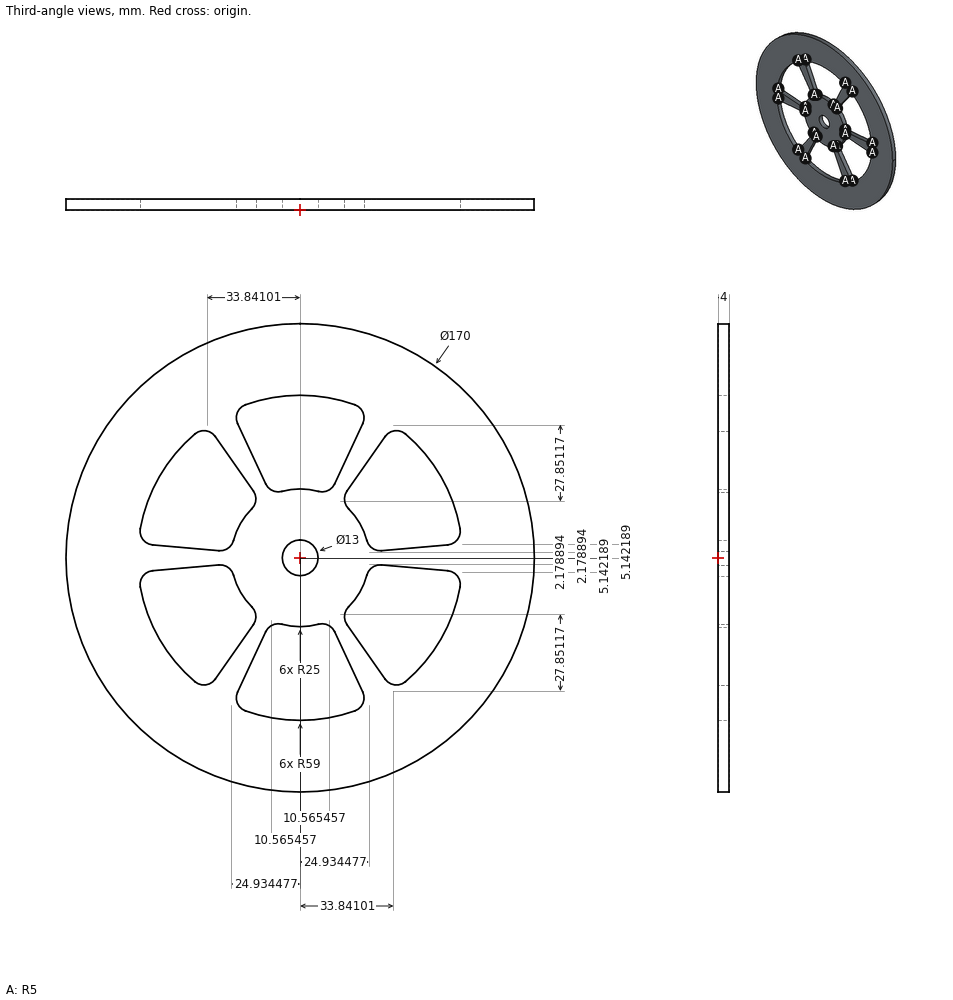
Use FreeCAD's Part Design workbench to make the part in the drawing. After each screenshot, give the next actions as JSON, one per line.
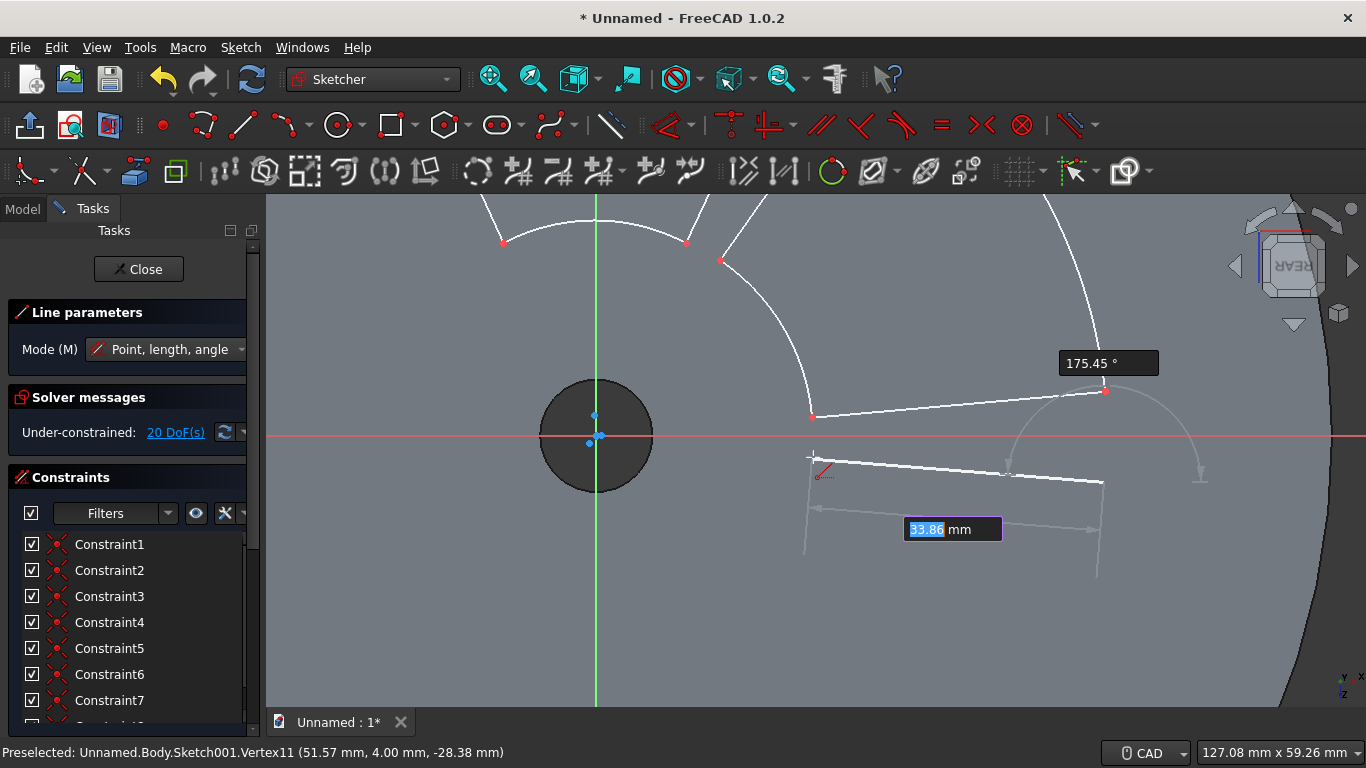
{"action": "left_click", "coordinate": [812, 455]}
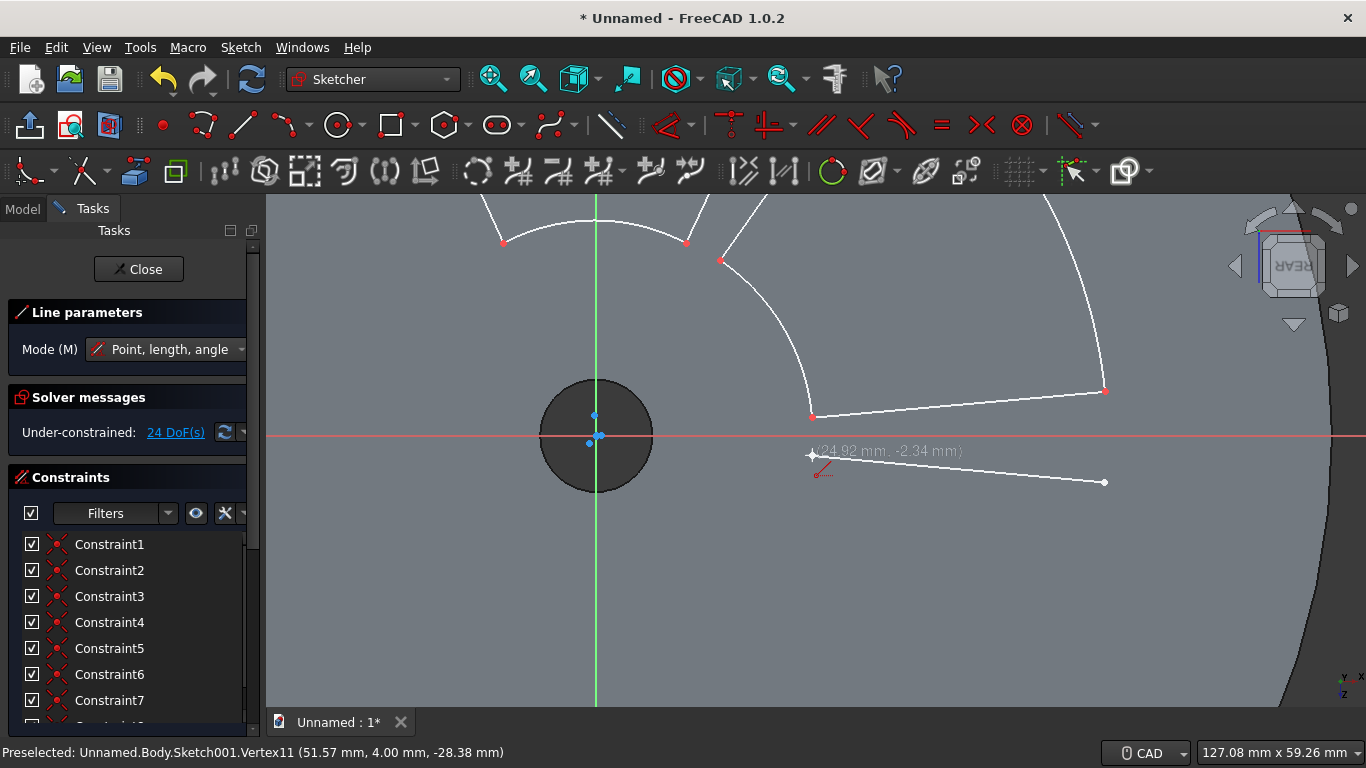
{"action": "scroll", "coordinate": [813, 457], "scroll_direction": "down", "scroll_amount": 6}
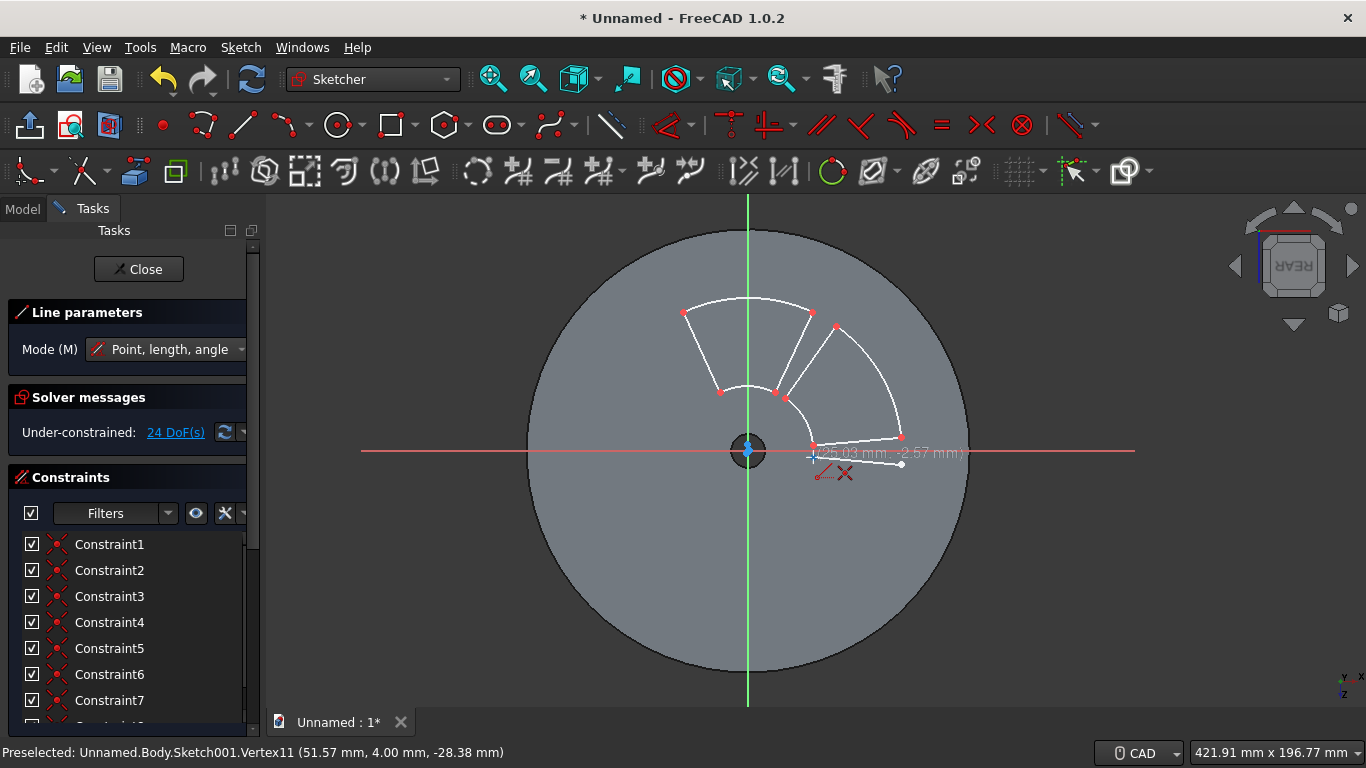
{"action": "left_click", "coordinate": [785, 504]}
{"action": "left_click", "coordinate": [836, 577]}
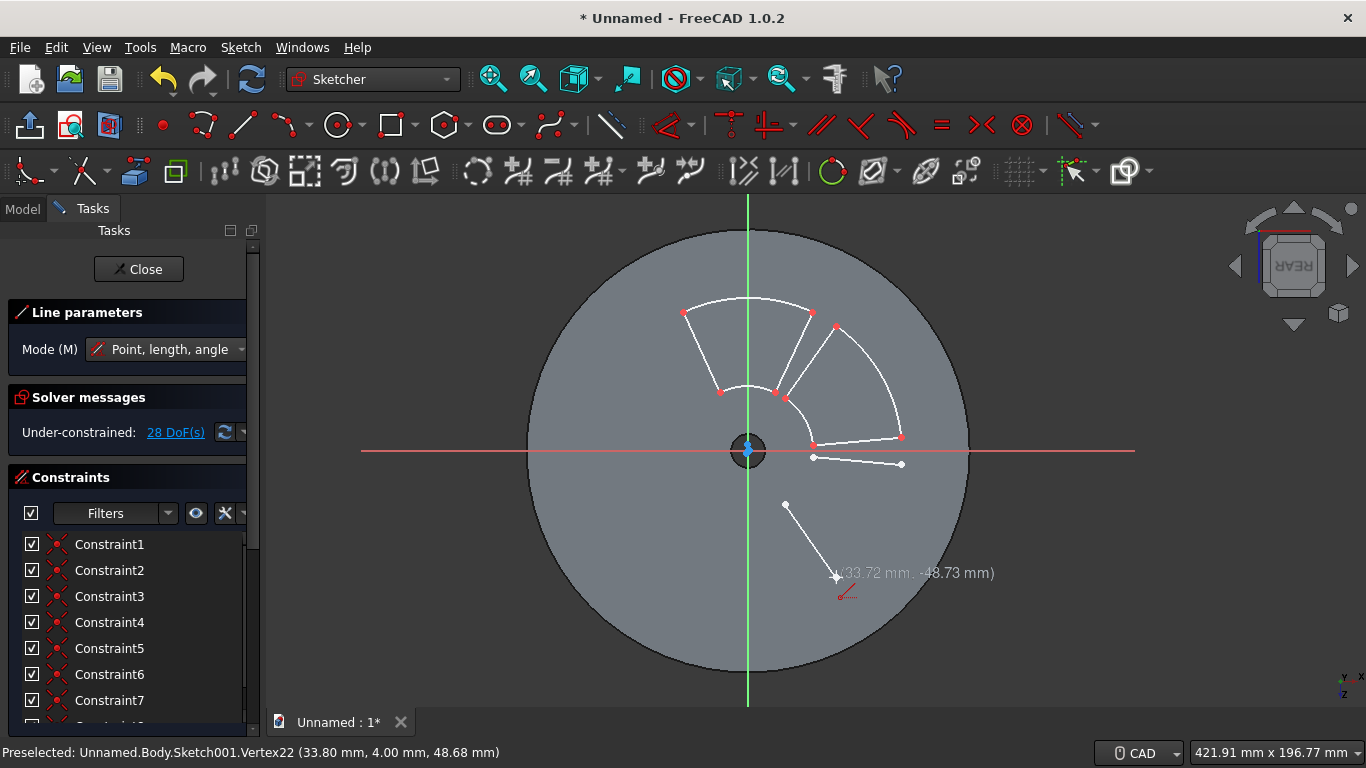
{"action": "left_click", "coordinate": [284, 126]}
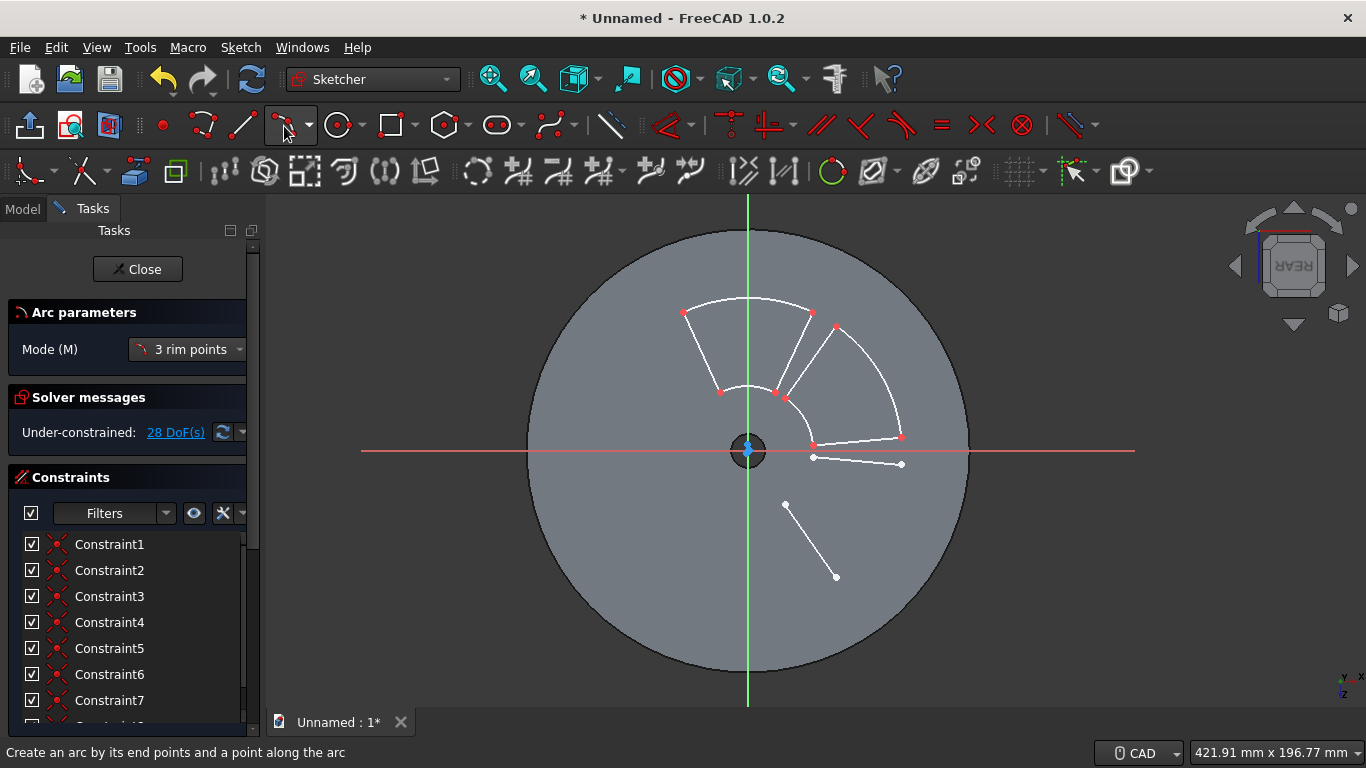
{"action": "scroll", "coordinate": [813, 457], "scroll_direction": "up", "scroll_amount": 6}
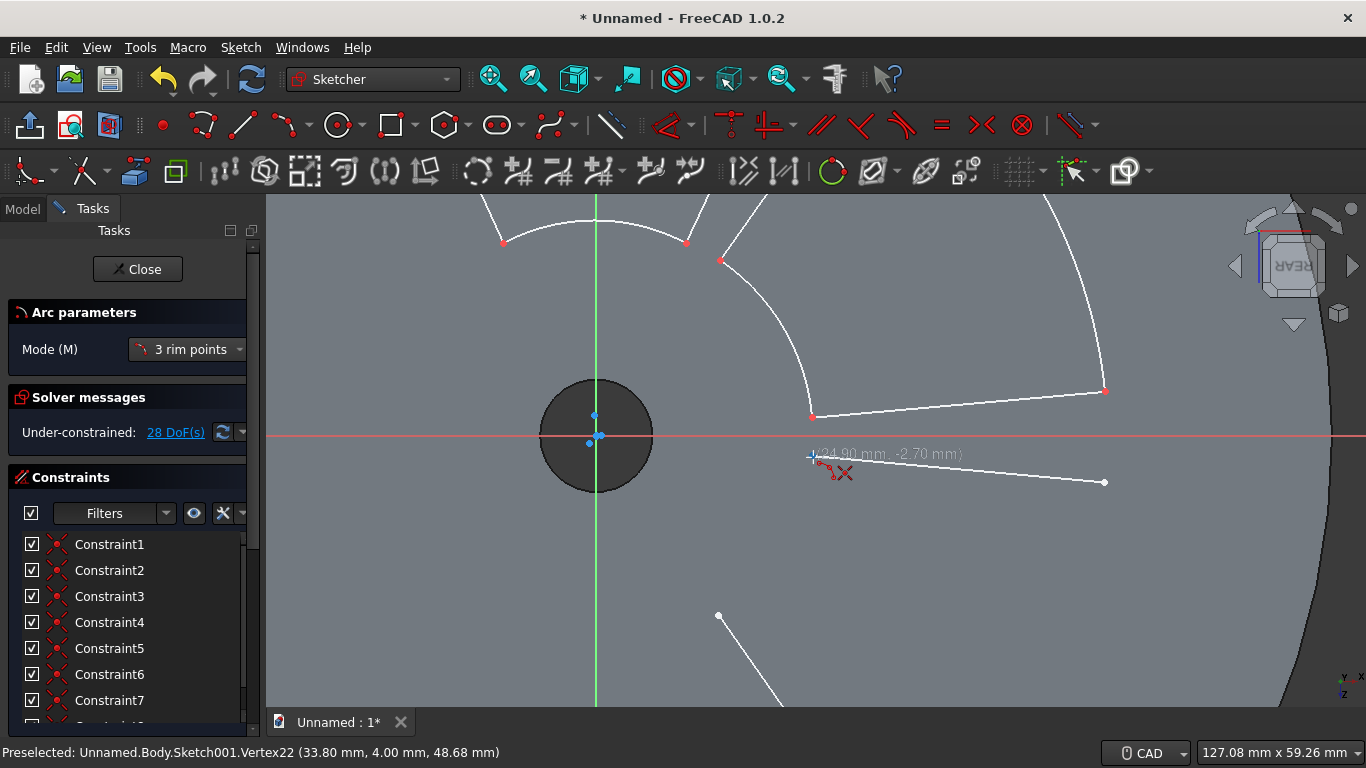
{"action": "left_click", "coordinate": [812, 456]}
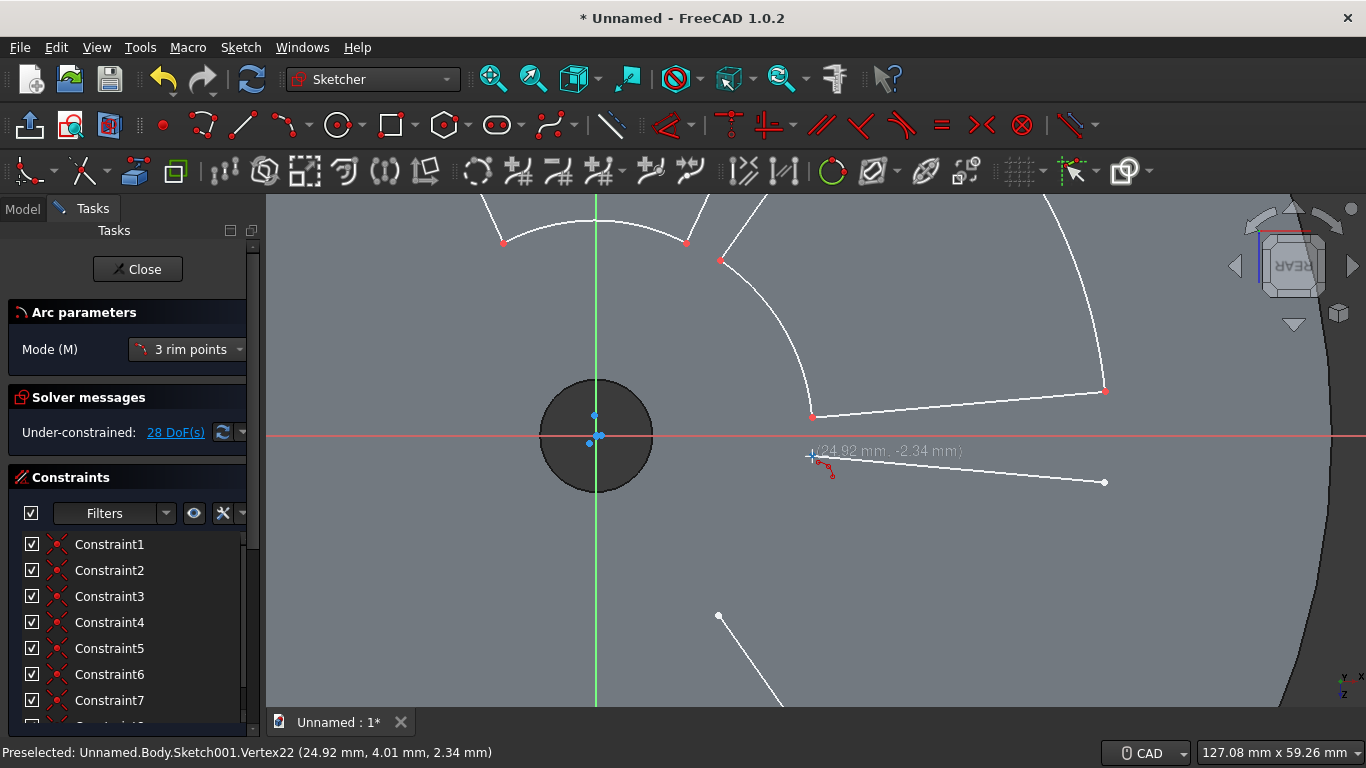
{"action": "scroll", "coordinate": [813, 457], "scroll_direction": "down", "scroll_amount": 6}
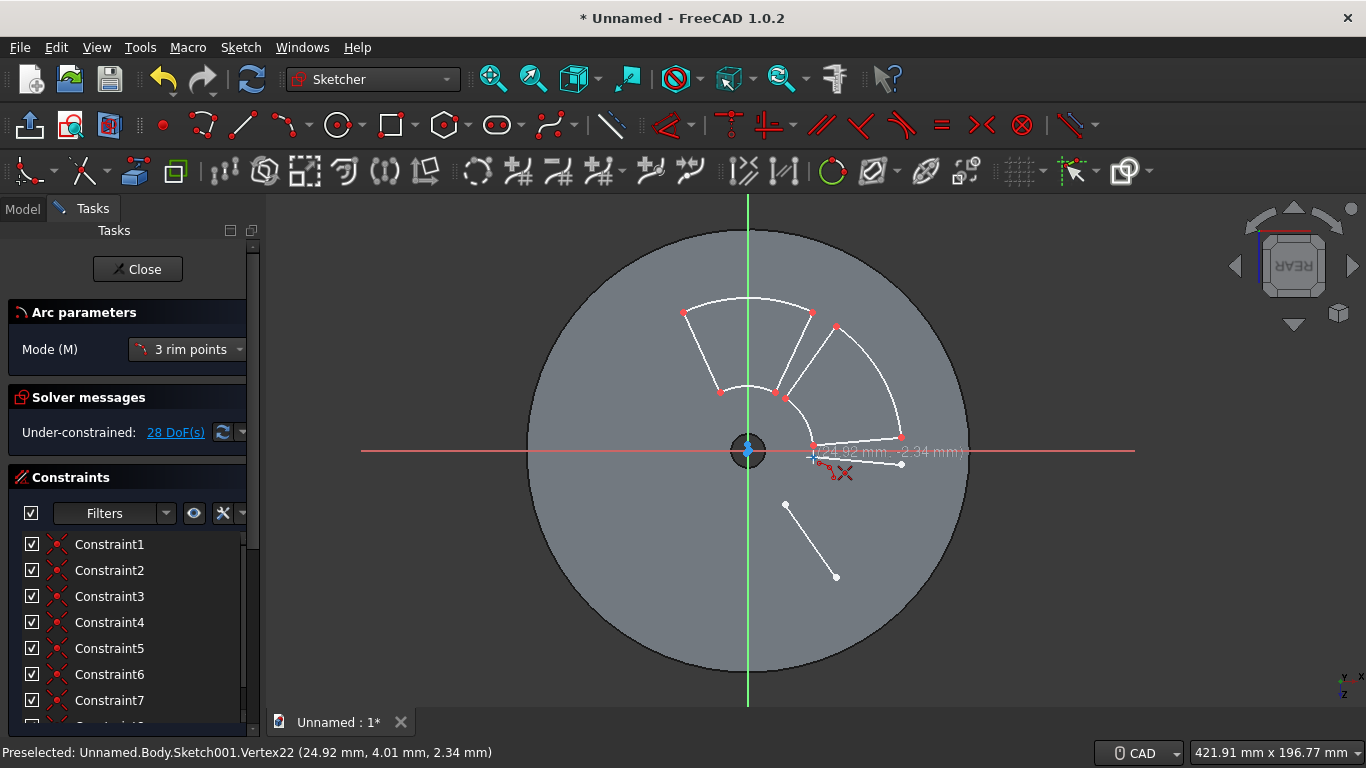
{"action": "left_click", "coordinate": [785, 505]}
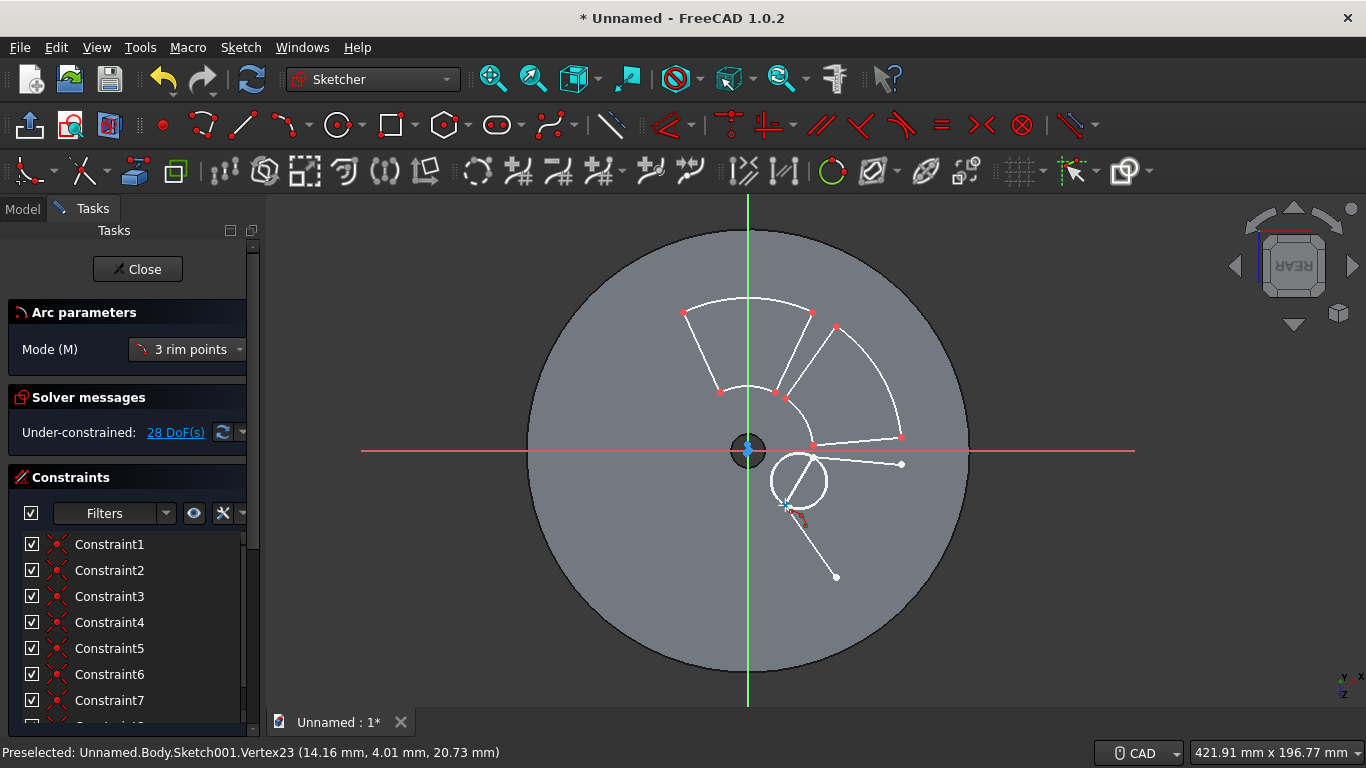
{"action": "scroll", "coordinate": [805, 484], "scroll_direction": "up", "scroll_amount": 5}